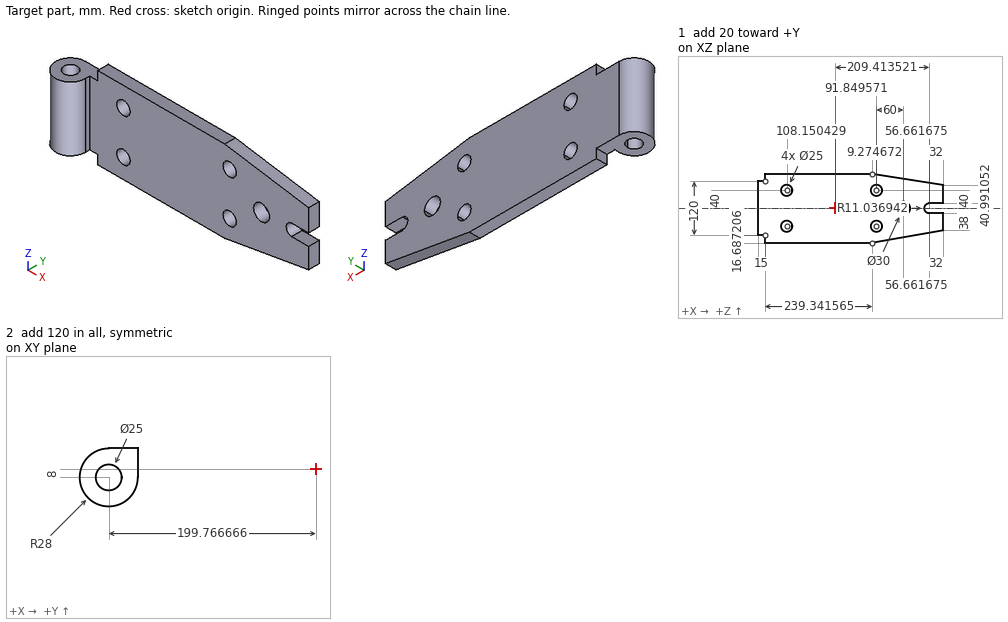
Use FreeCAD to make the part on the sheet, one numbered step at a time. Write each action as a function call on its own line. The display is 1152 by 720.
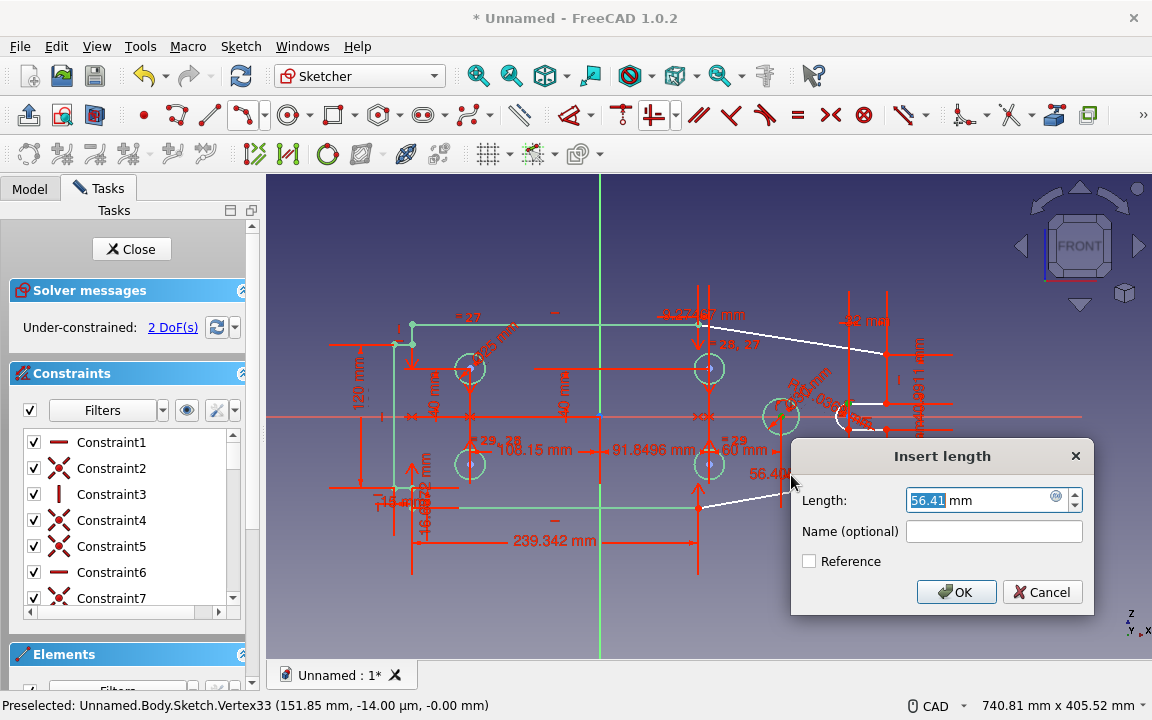
text(56.661675)
key(Return)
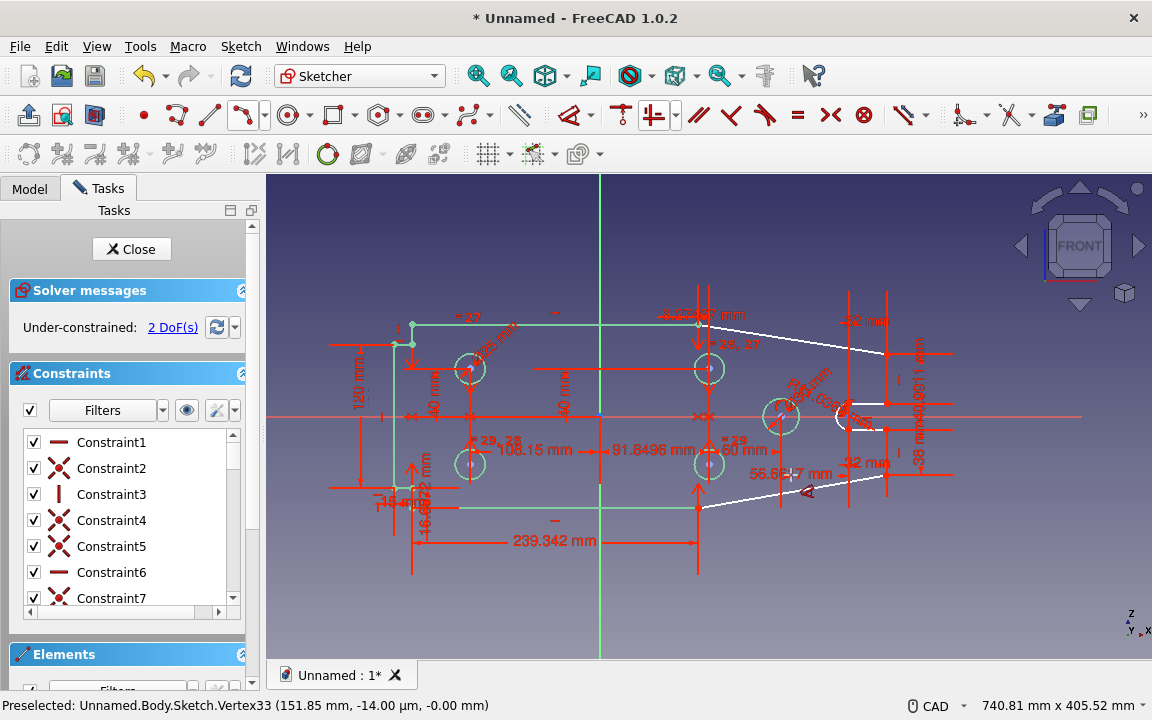
click(849, 430)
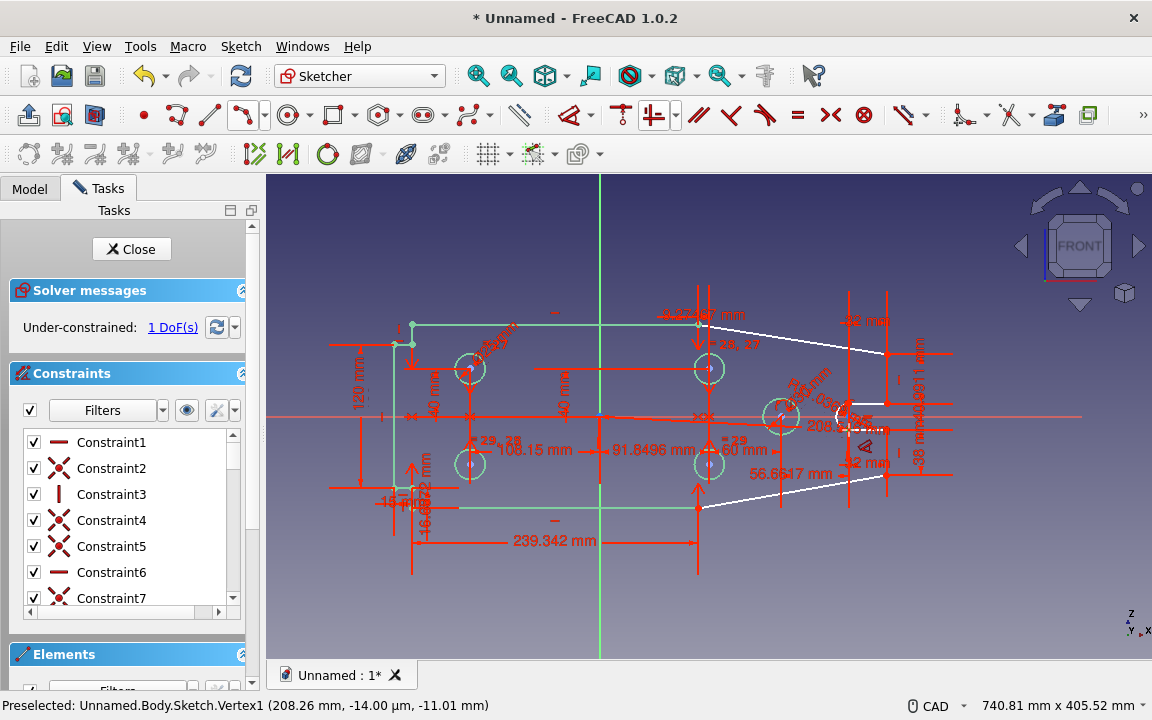
click(781, 417)
click(815, 359)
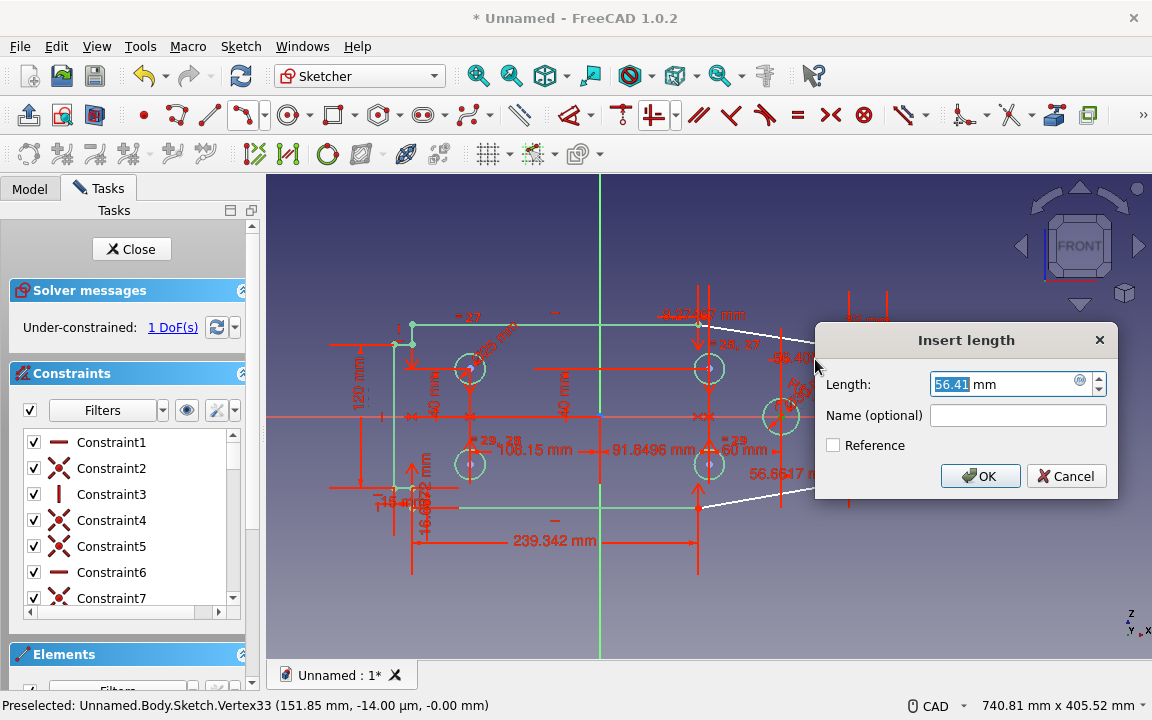
text(56.661675)
key(Return)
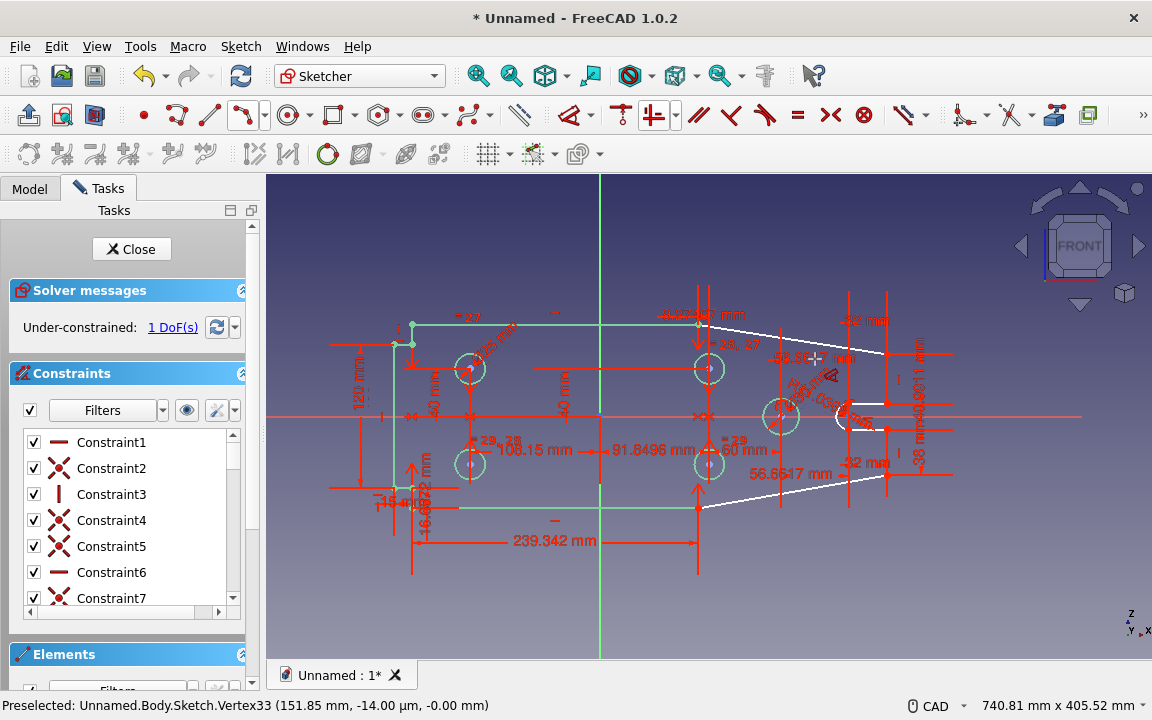
click(850, 417)
click(667, 383)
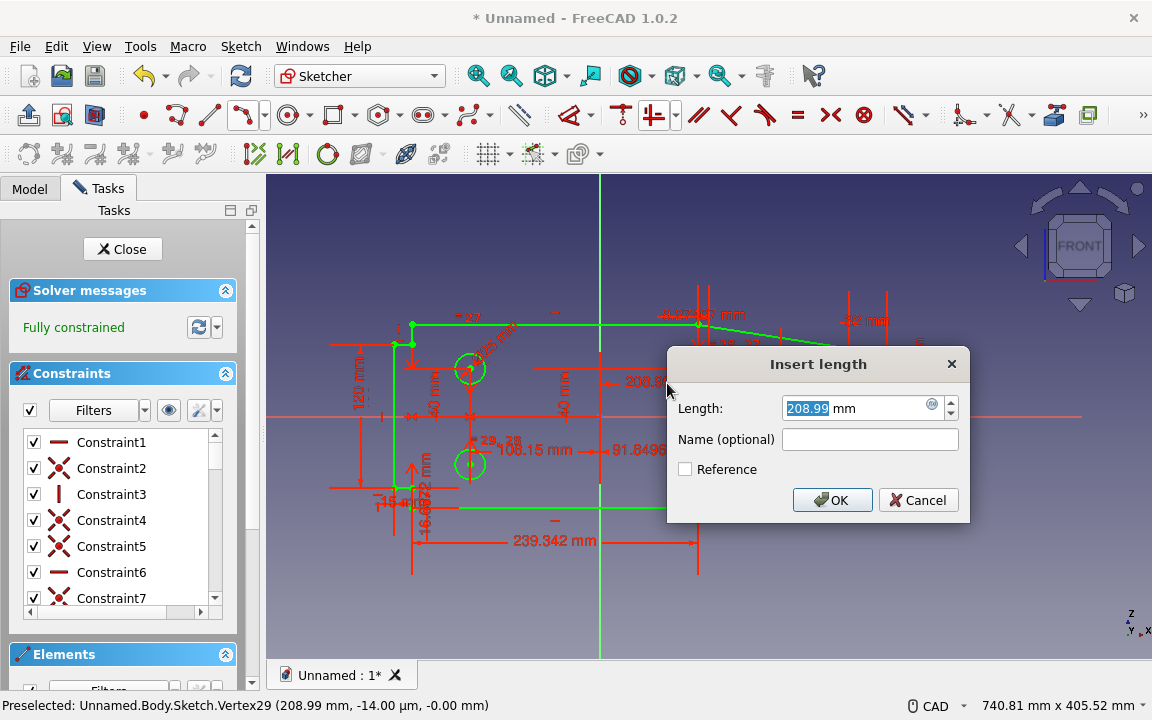
text(209.413521)
key(Return)
key(Escape)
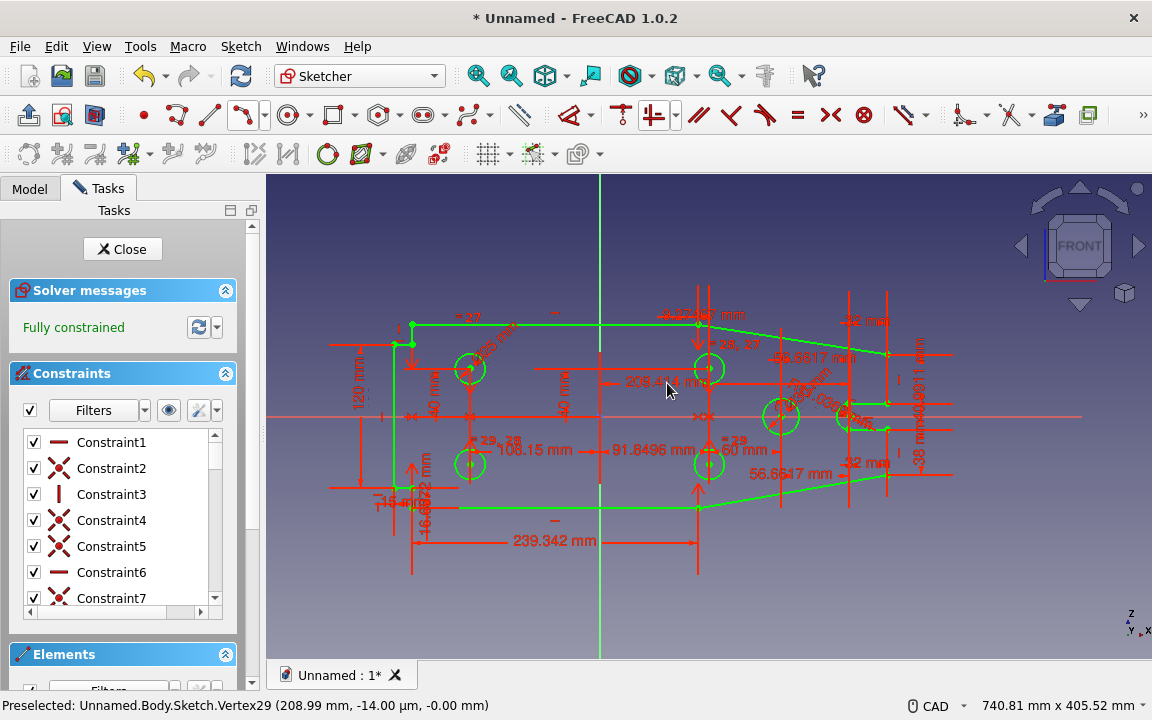
click(123, 249)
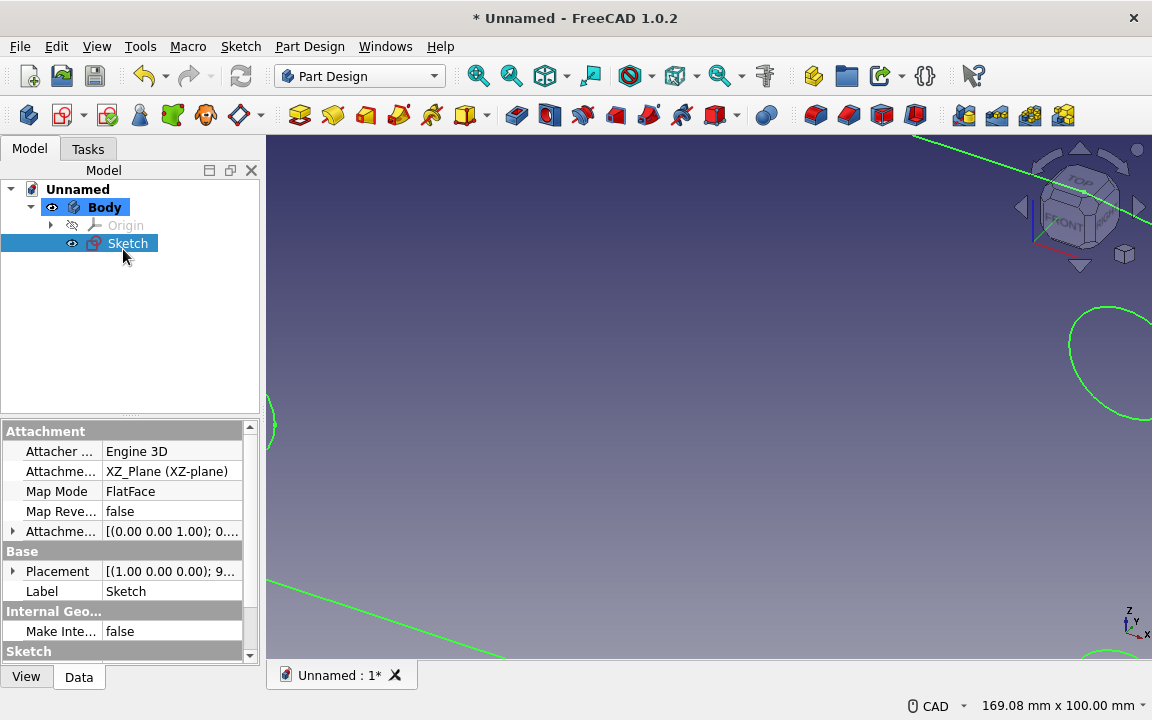
click(300, 116)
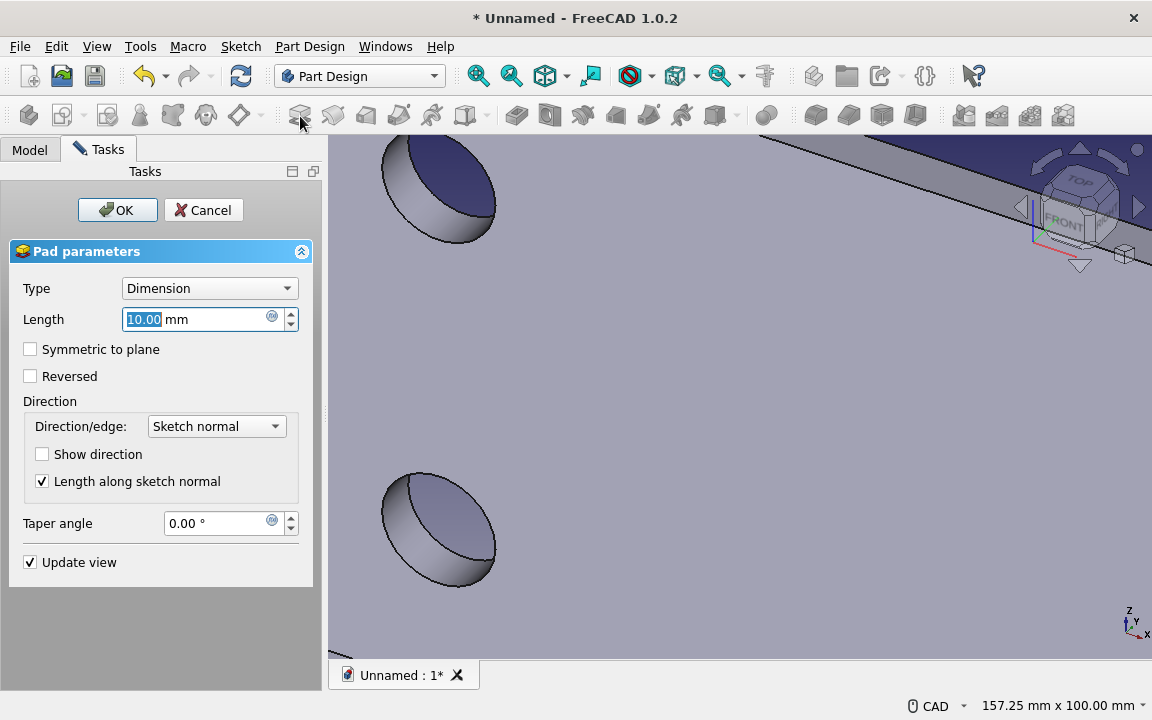
text(20)
key(Tab)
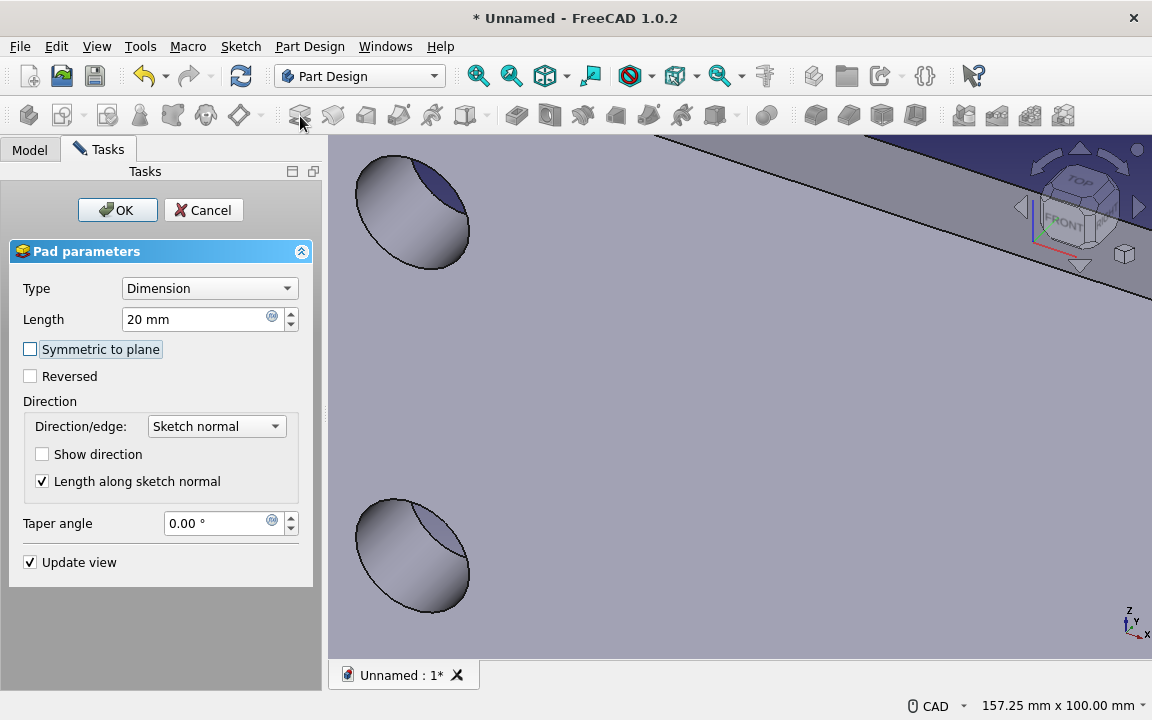
click(31, 376)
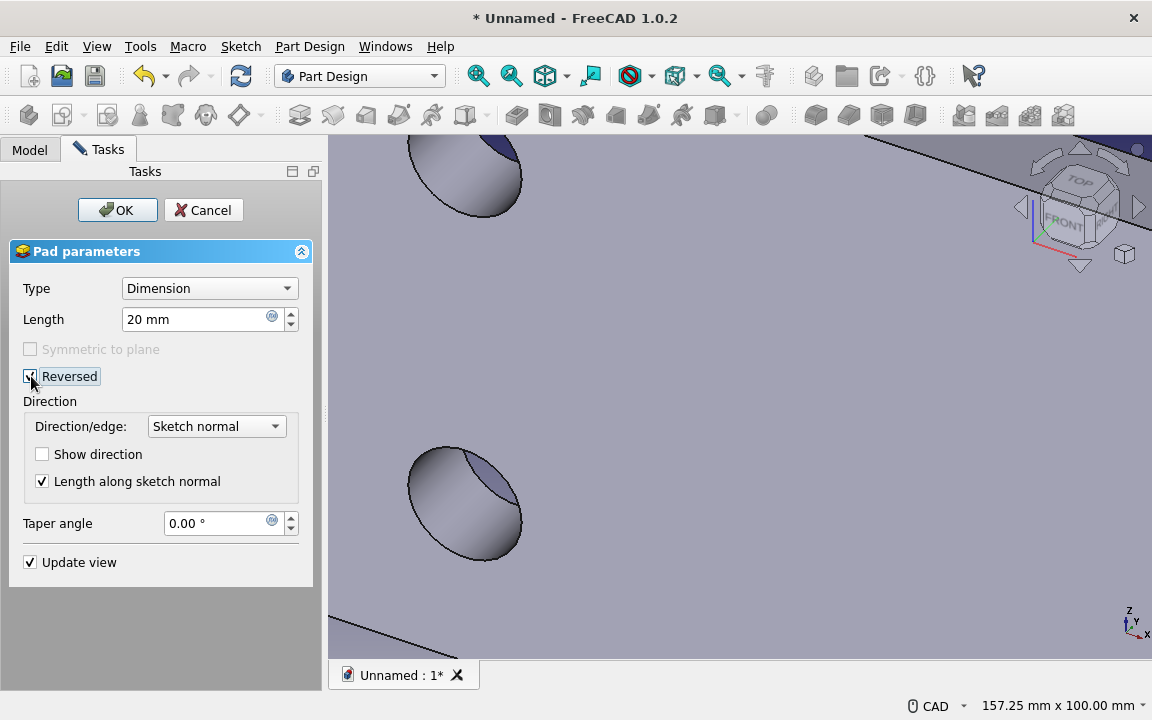
click(118, 210)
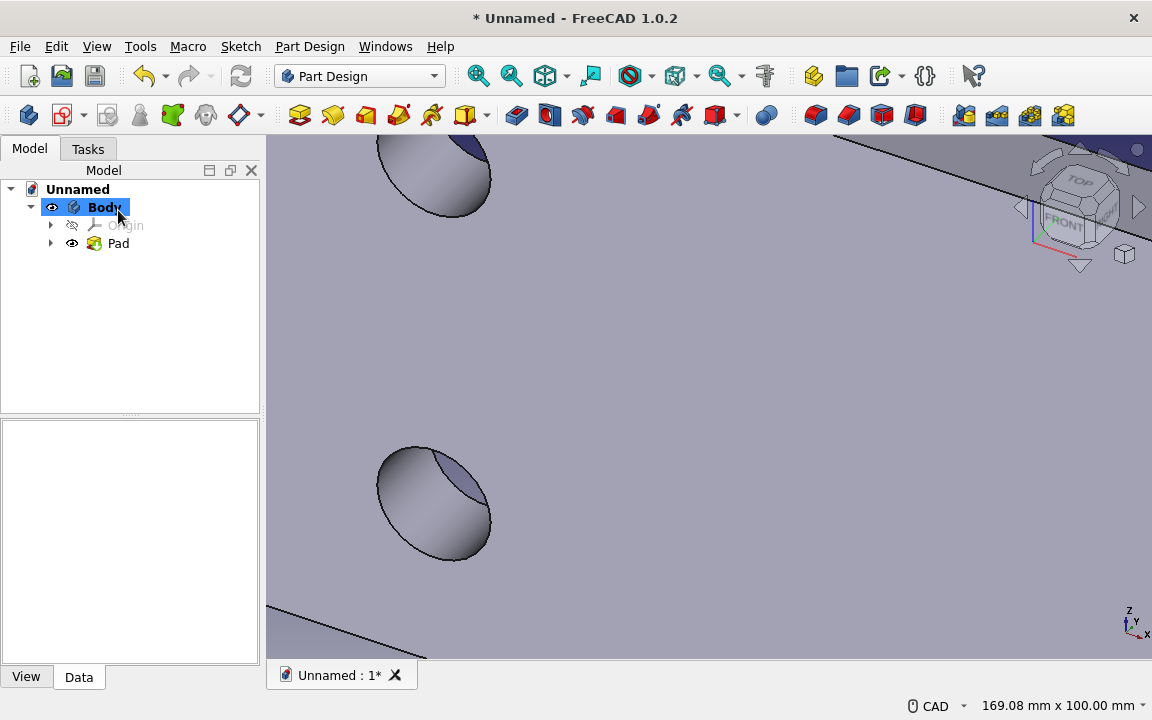
click(479, 76)